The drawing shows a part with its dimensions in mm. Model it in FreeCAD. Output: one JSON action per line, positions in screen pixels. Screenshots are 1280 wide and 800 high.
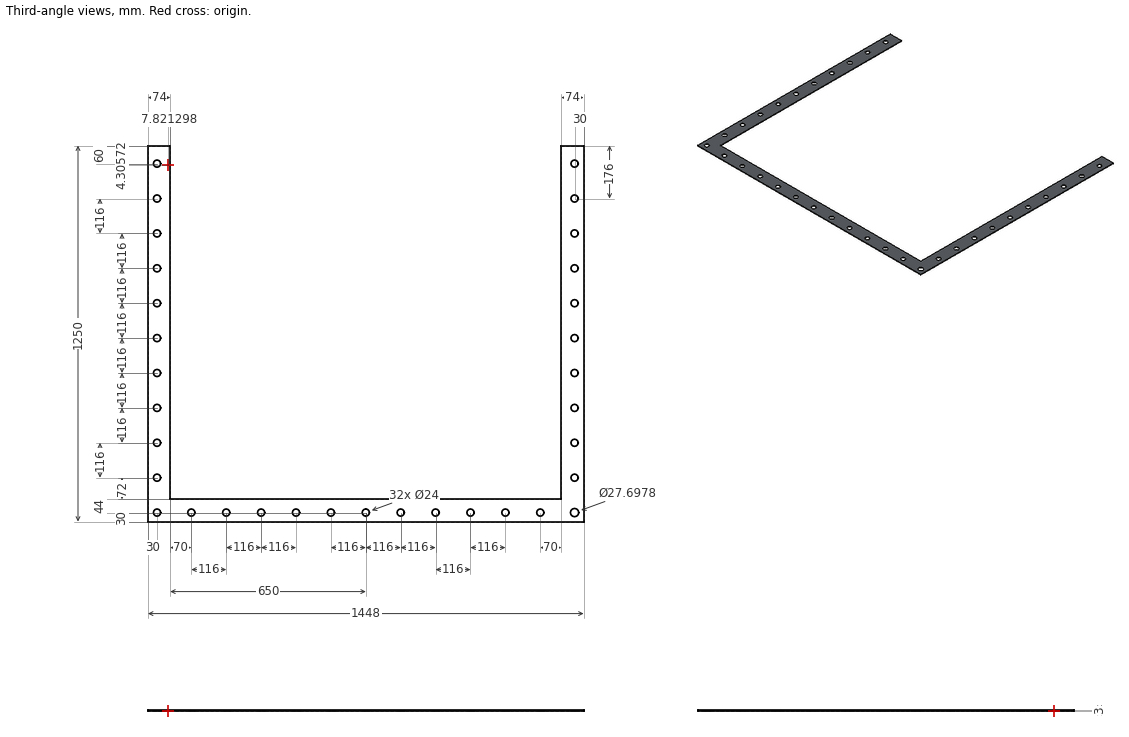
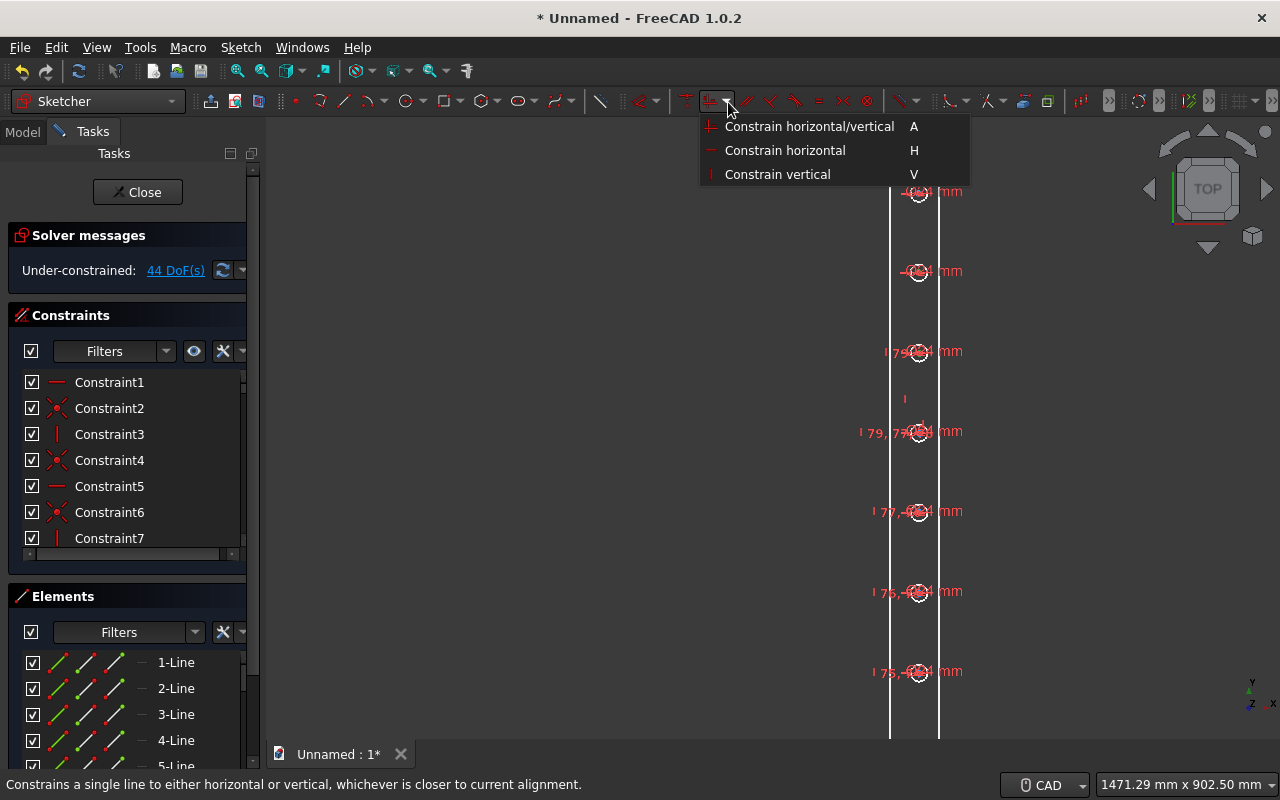
{"action": "left_click", "coordinate": [835, 174]}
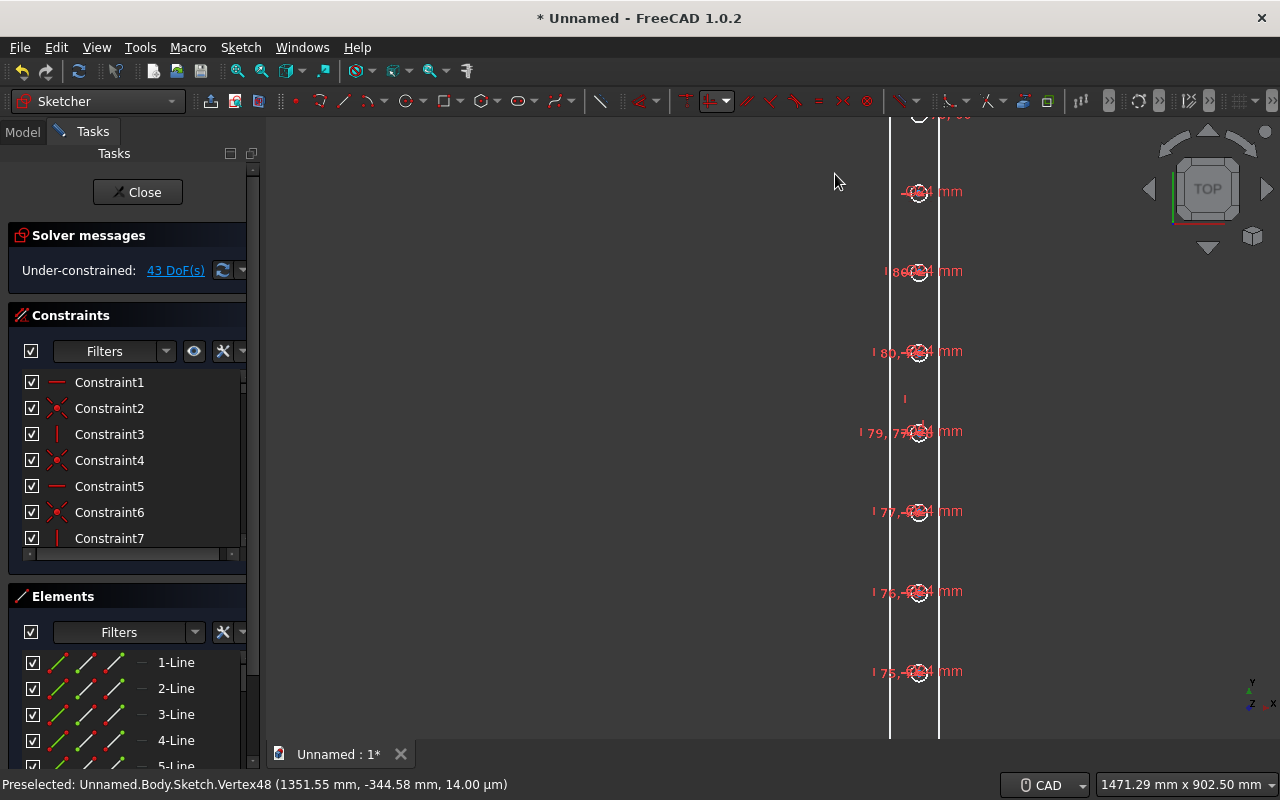
{"action": "left_click", "coordinate": [919, 273]}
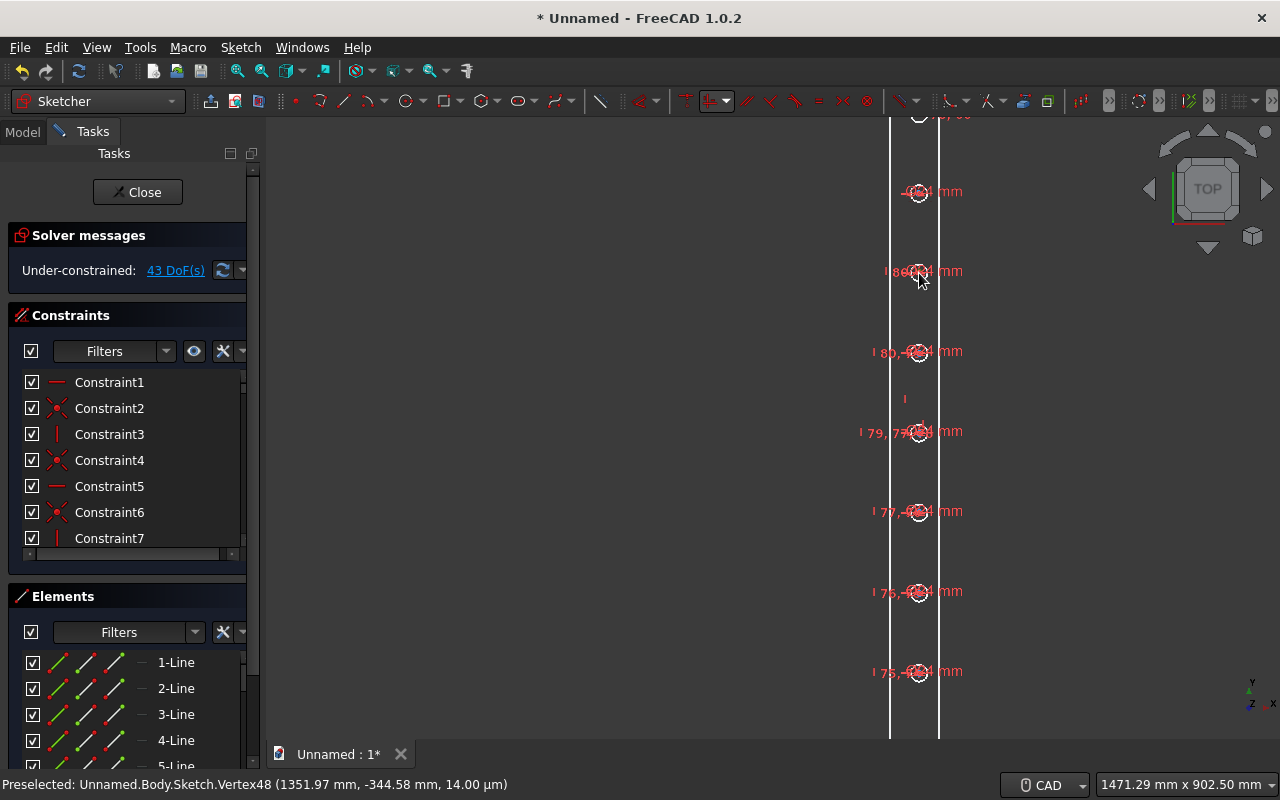
{"action": "left_click", "coordinate": [919, 194]}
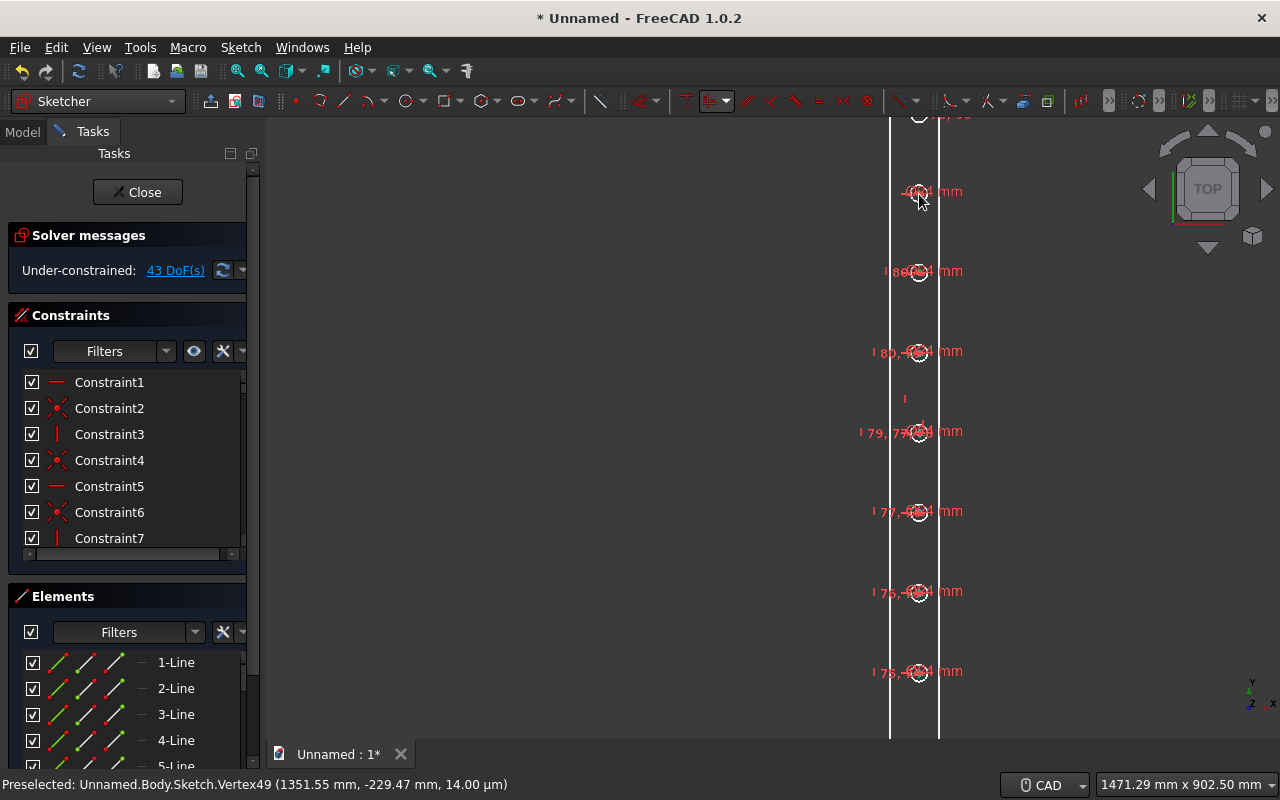
{"action": "left_click", "coordinate": [728, 102]}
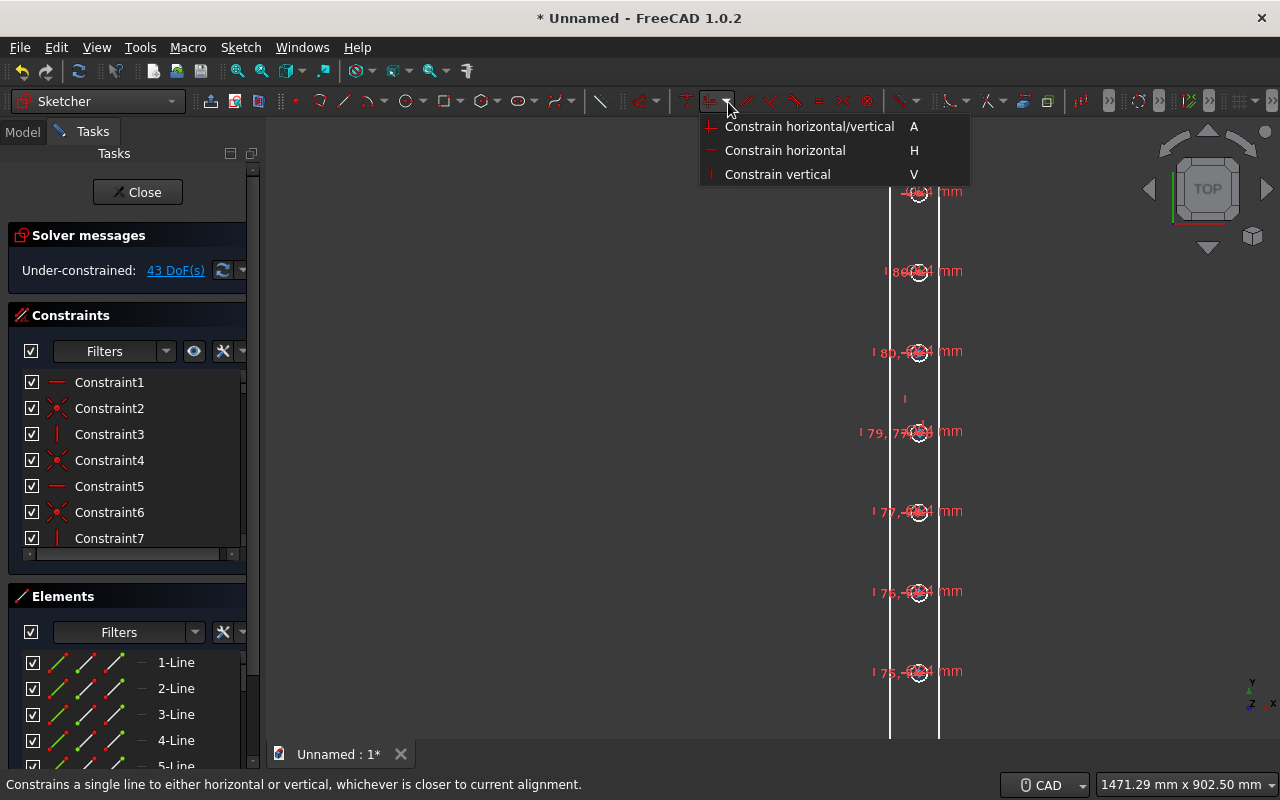
{"action": "left_click", "coordinate": [835, 174]}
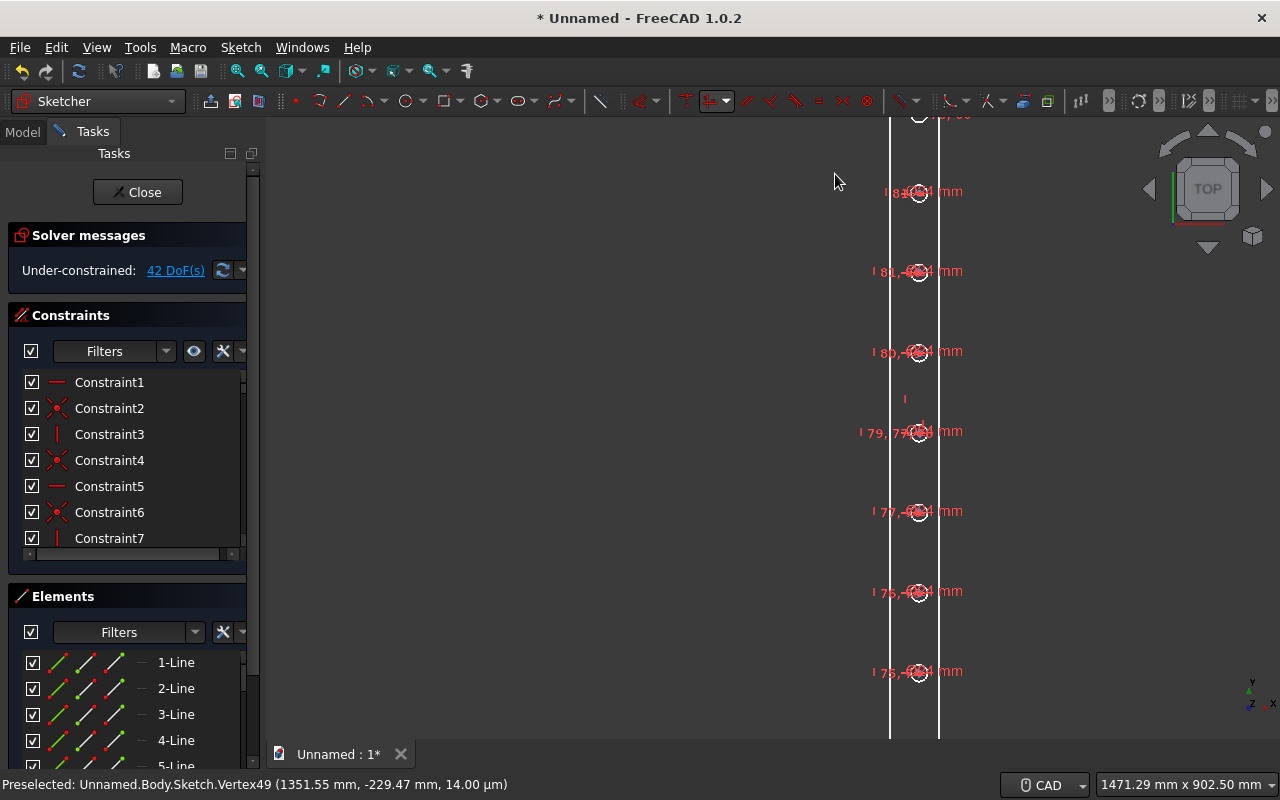
{"action": "scroll", "coordinate": [920, 433], "scroll_direction": "down", "scroll_amount": 4}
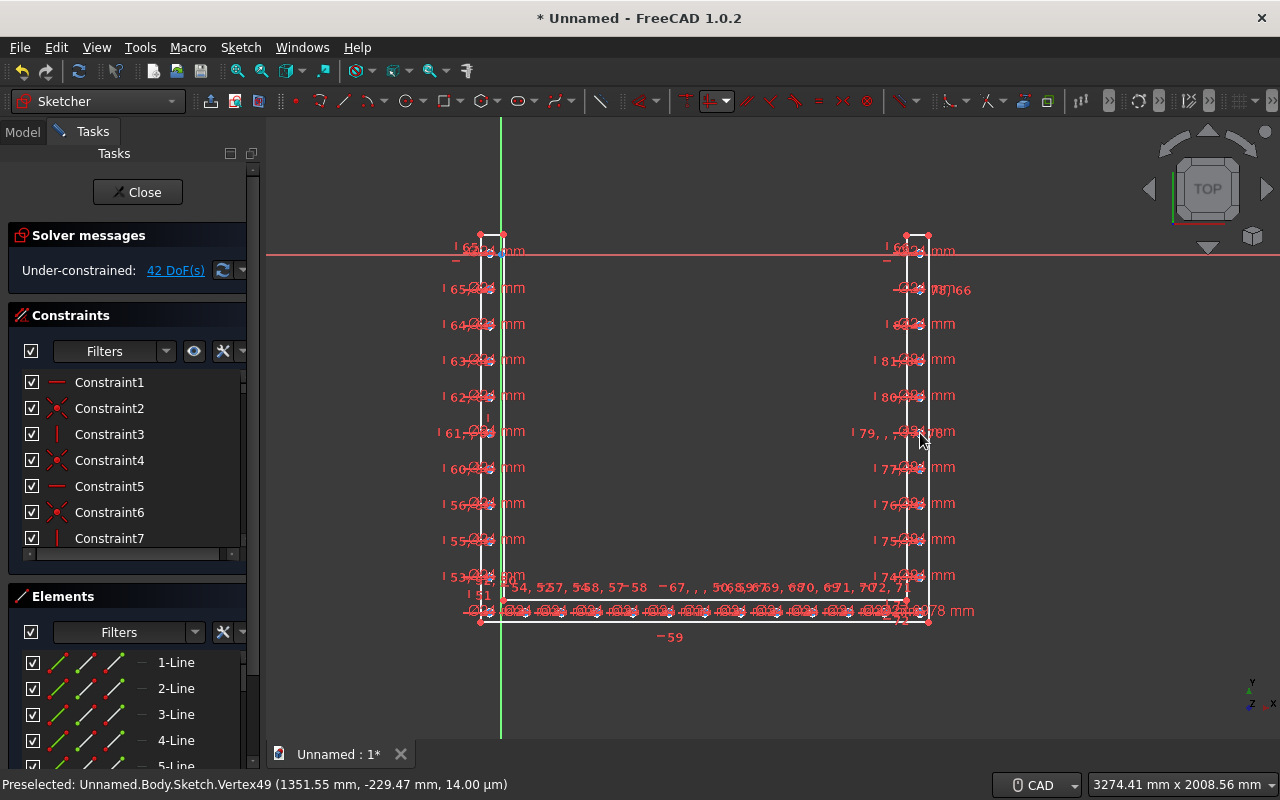
{"action": "scroll", "coordinate": [497, 235], "scroll_direction": "up", "scroll_amount": 6}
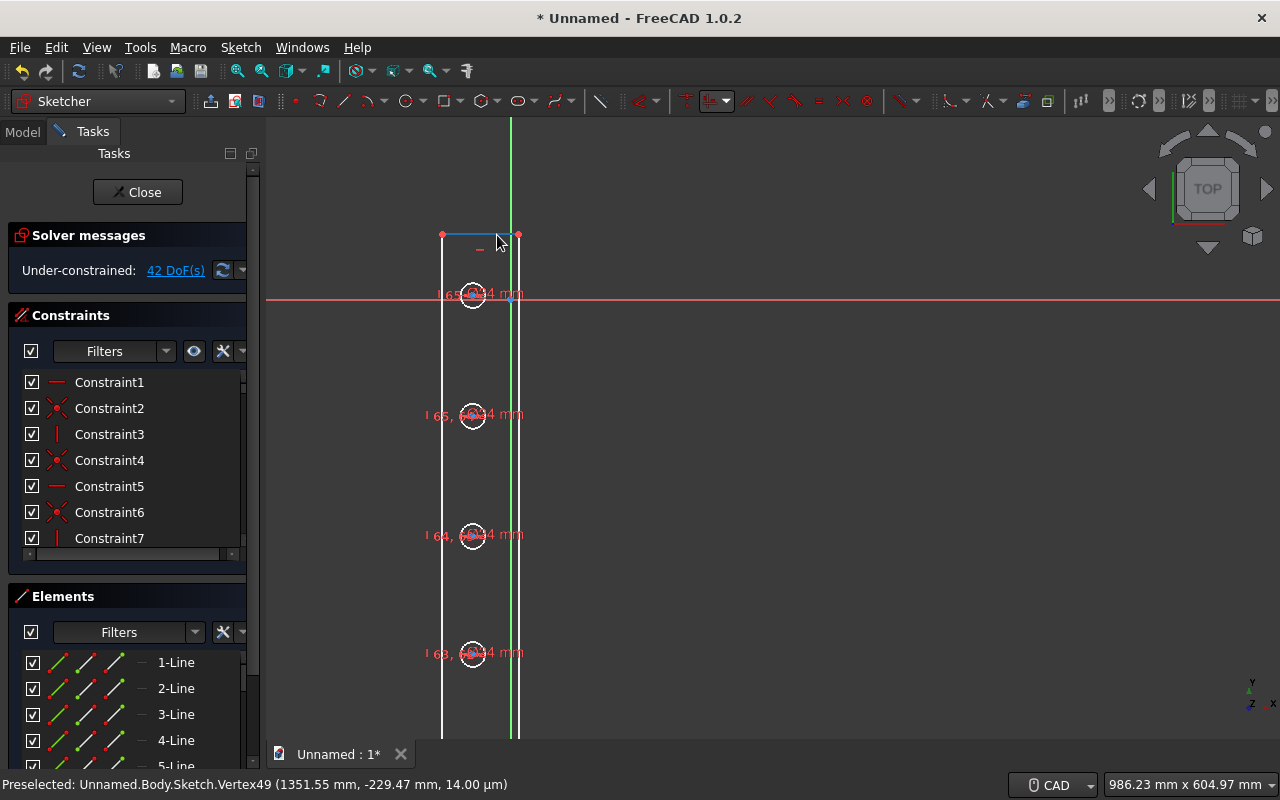
{"action": "left_click", "coordinate": [496, 234]}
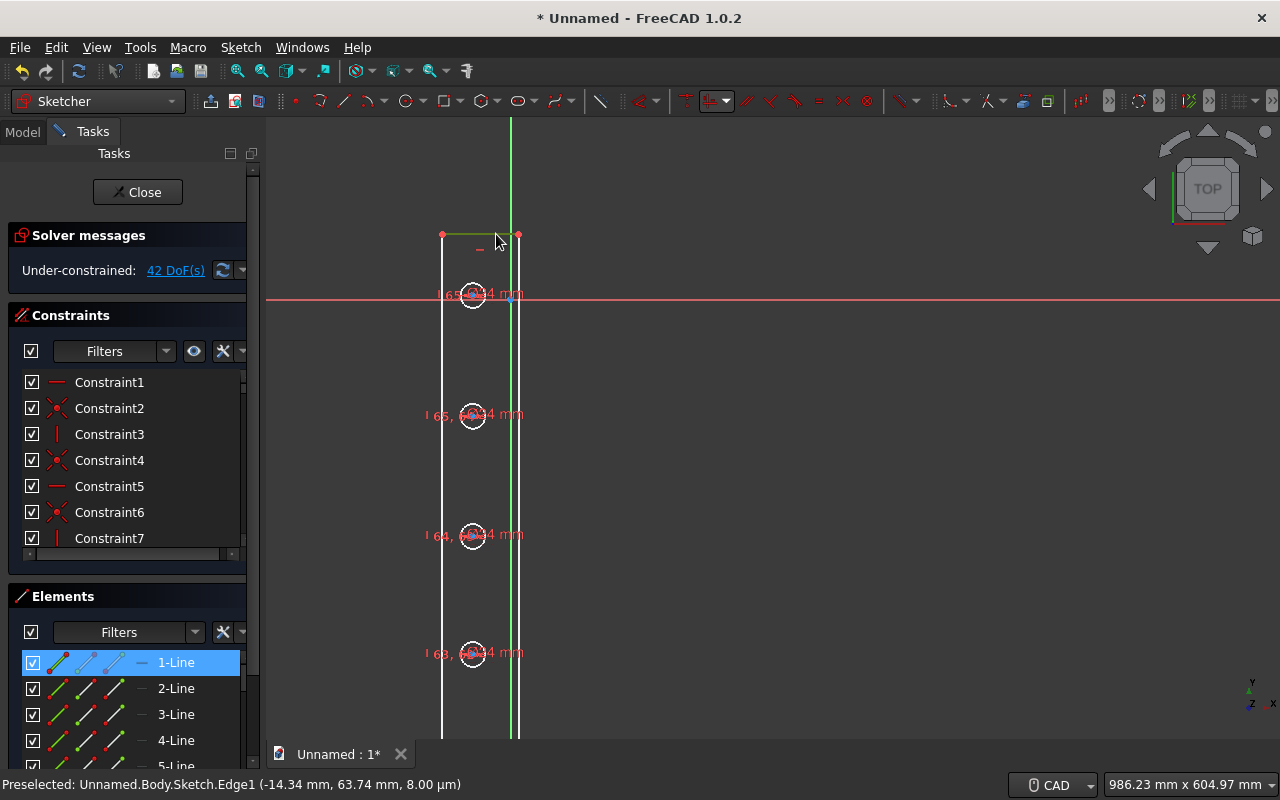
{"action": "left_click", "coordinate": [658, 102]}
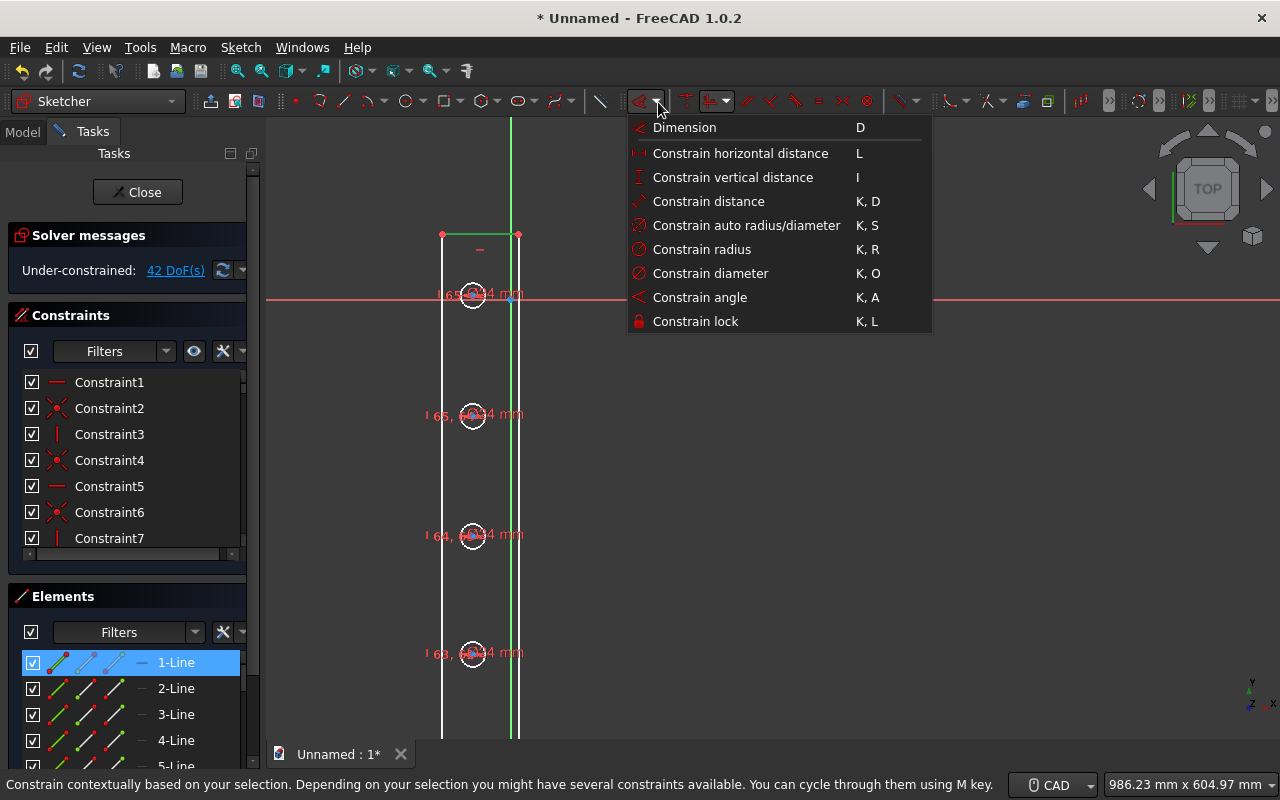
{"action": "left_click", "coordinate": [780, 153]}